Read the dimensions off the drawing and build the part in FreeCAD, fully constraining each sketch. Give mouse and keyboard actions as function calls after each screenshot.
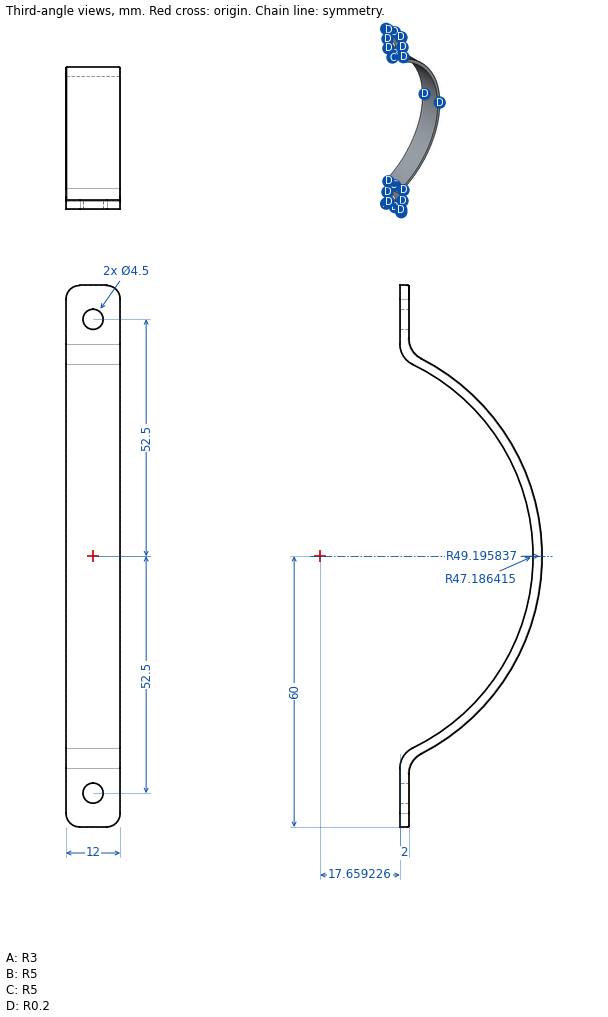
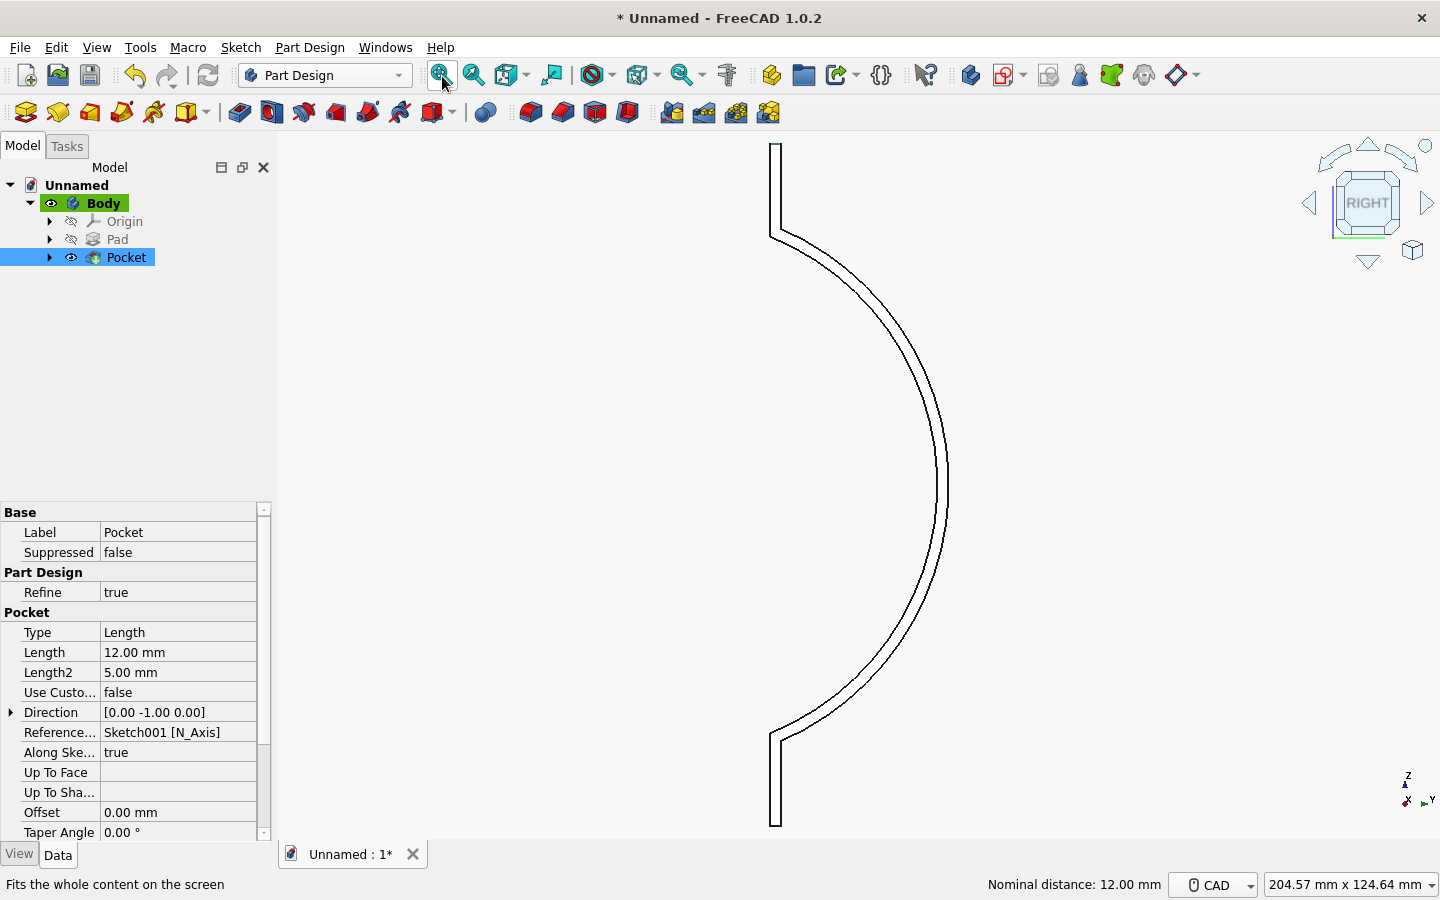
key(5)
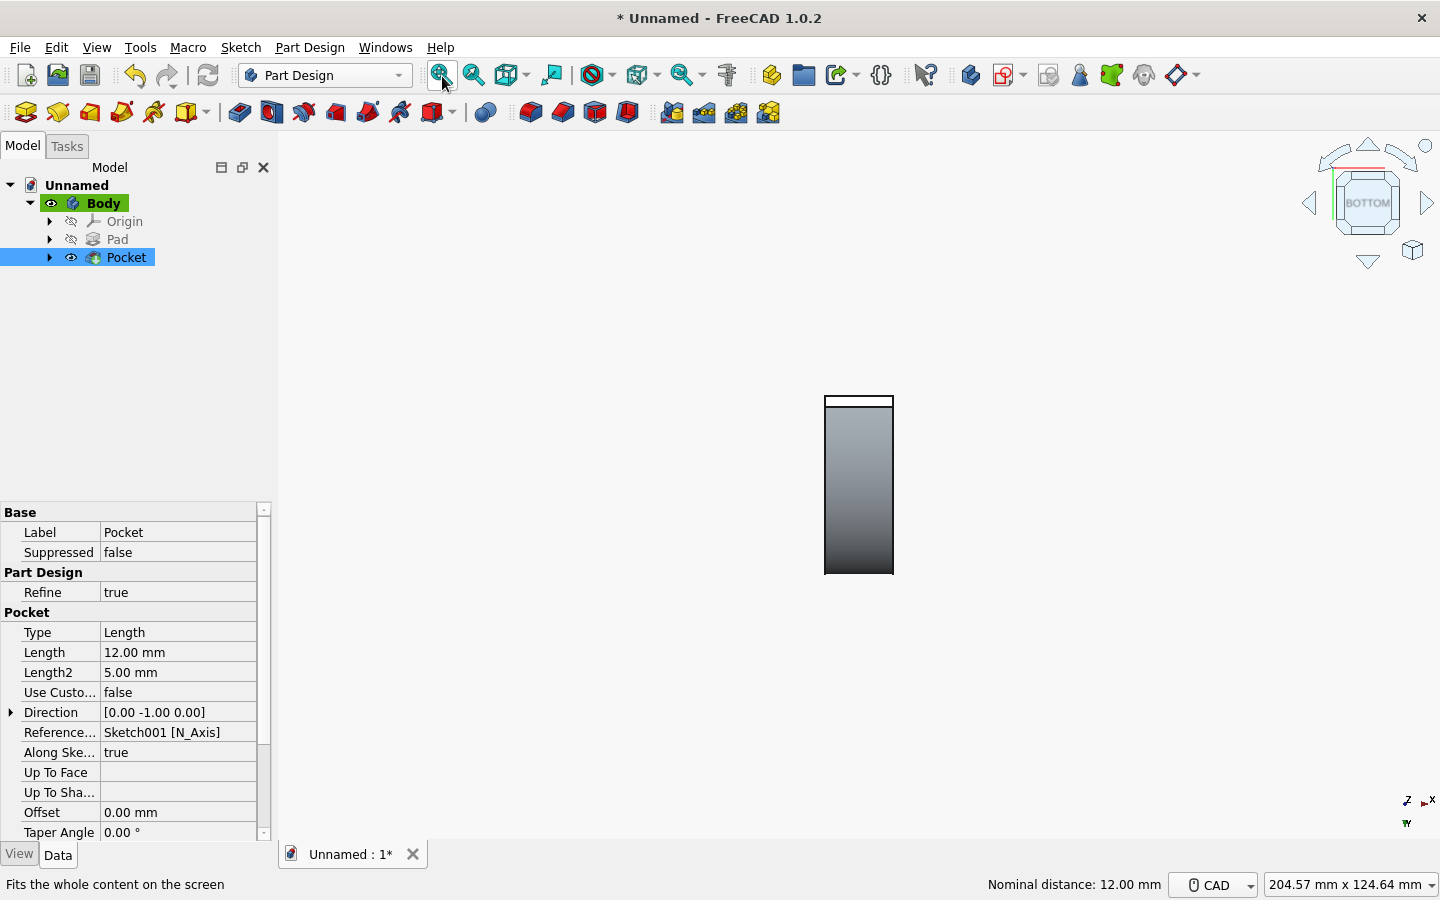
key(v)
key(f)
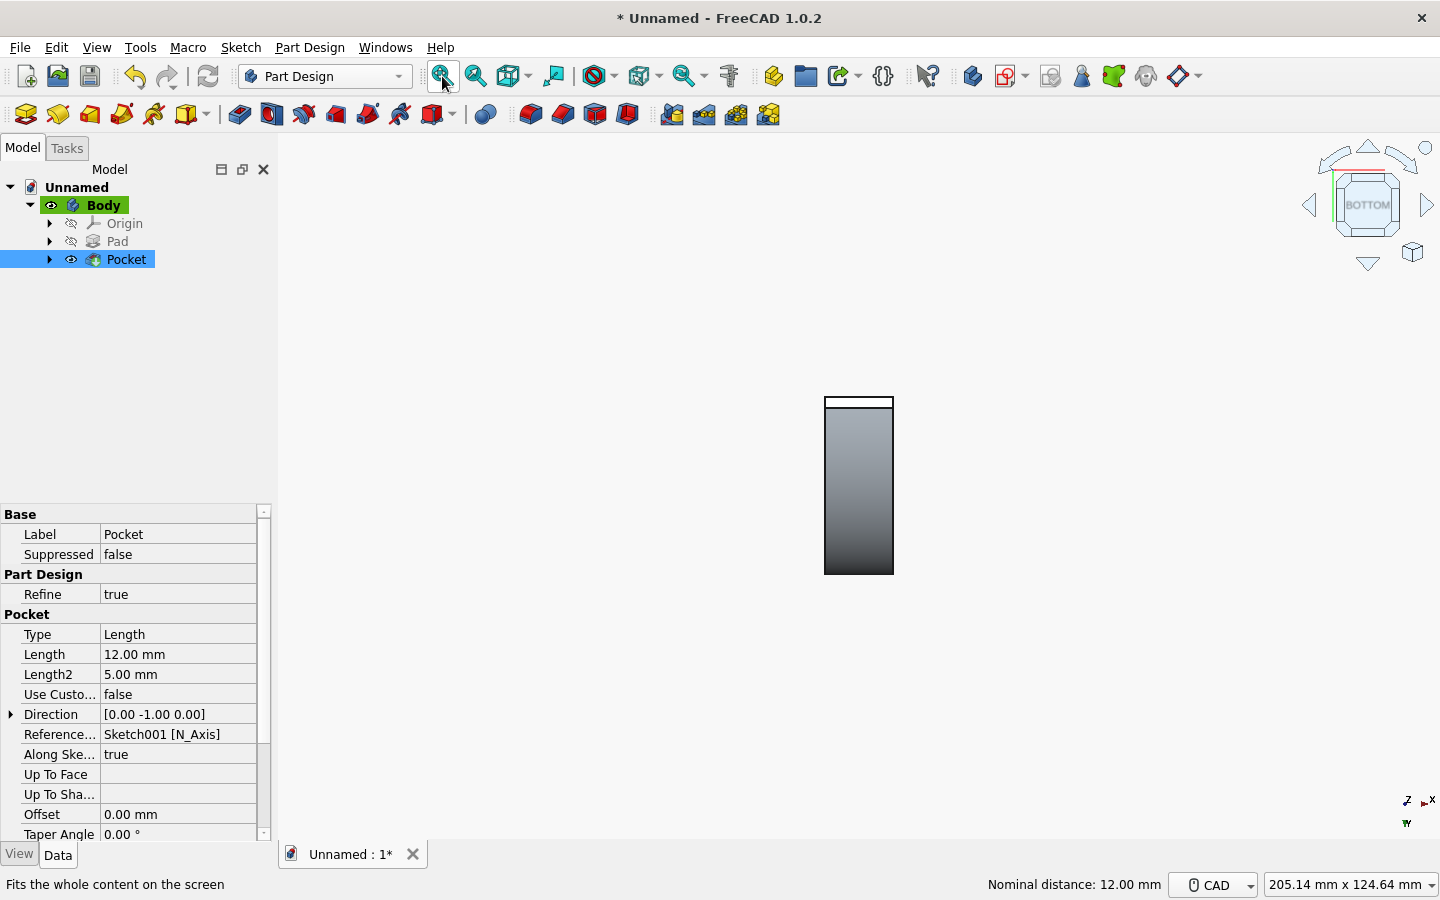
scroll(893, 401, up, 7)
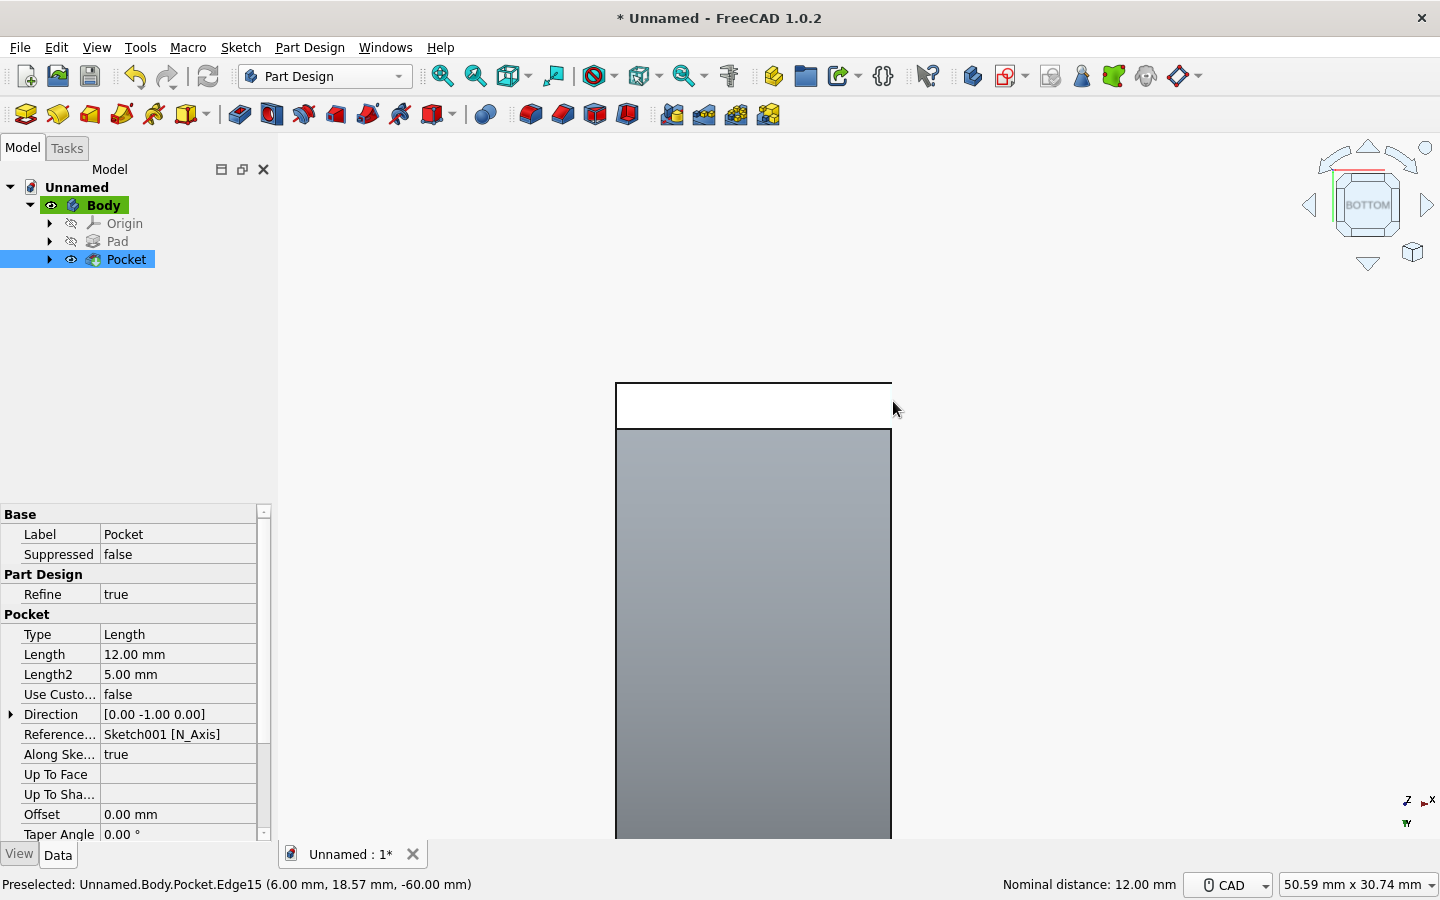
click(891, 405, ctrl)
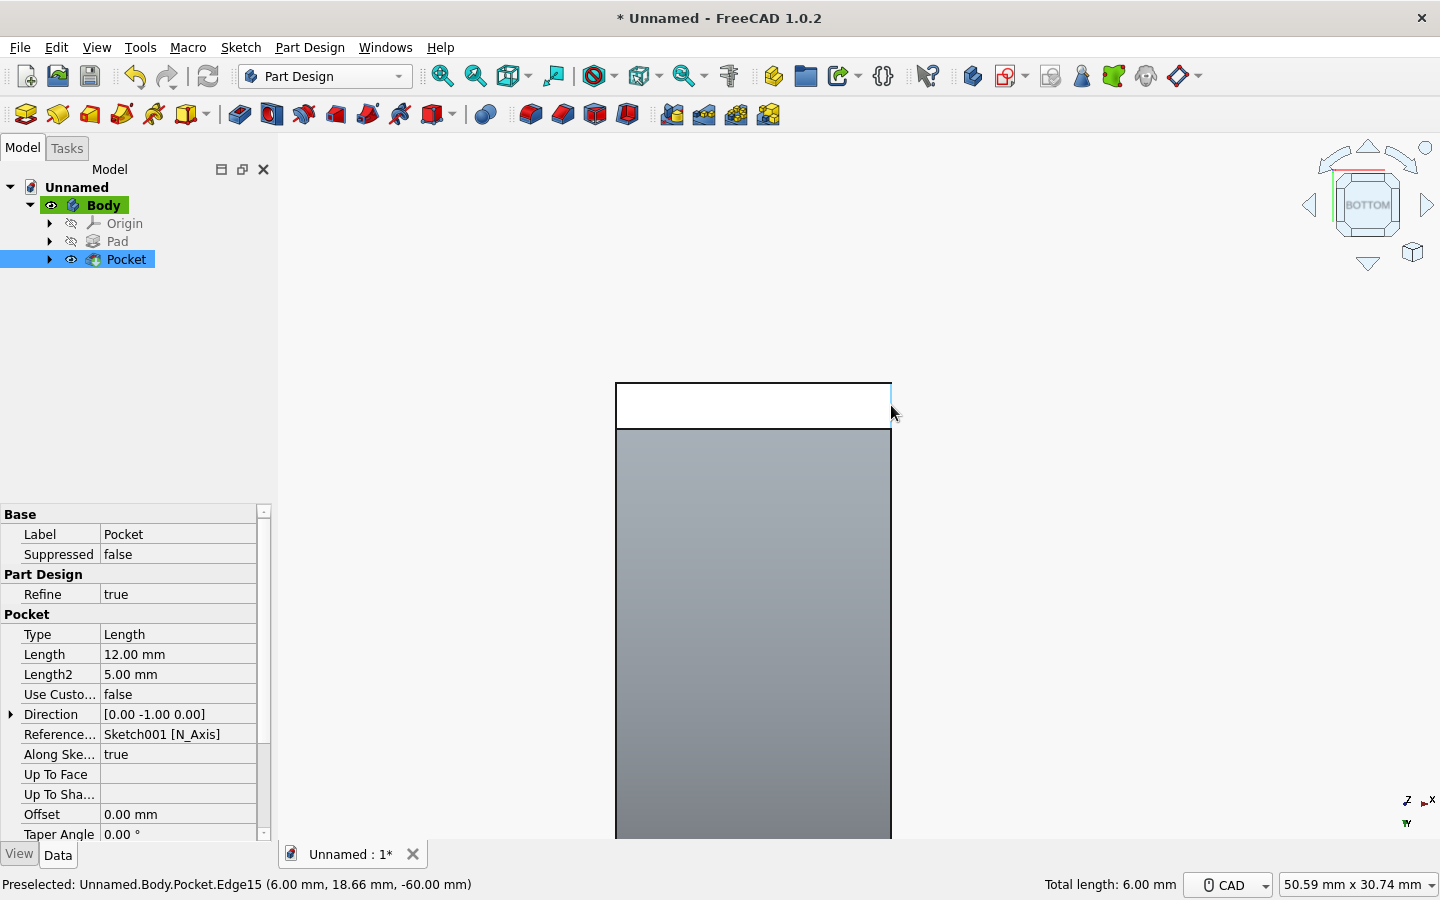
click(616, 405, ctrl)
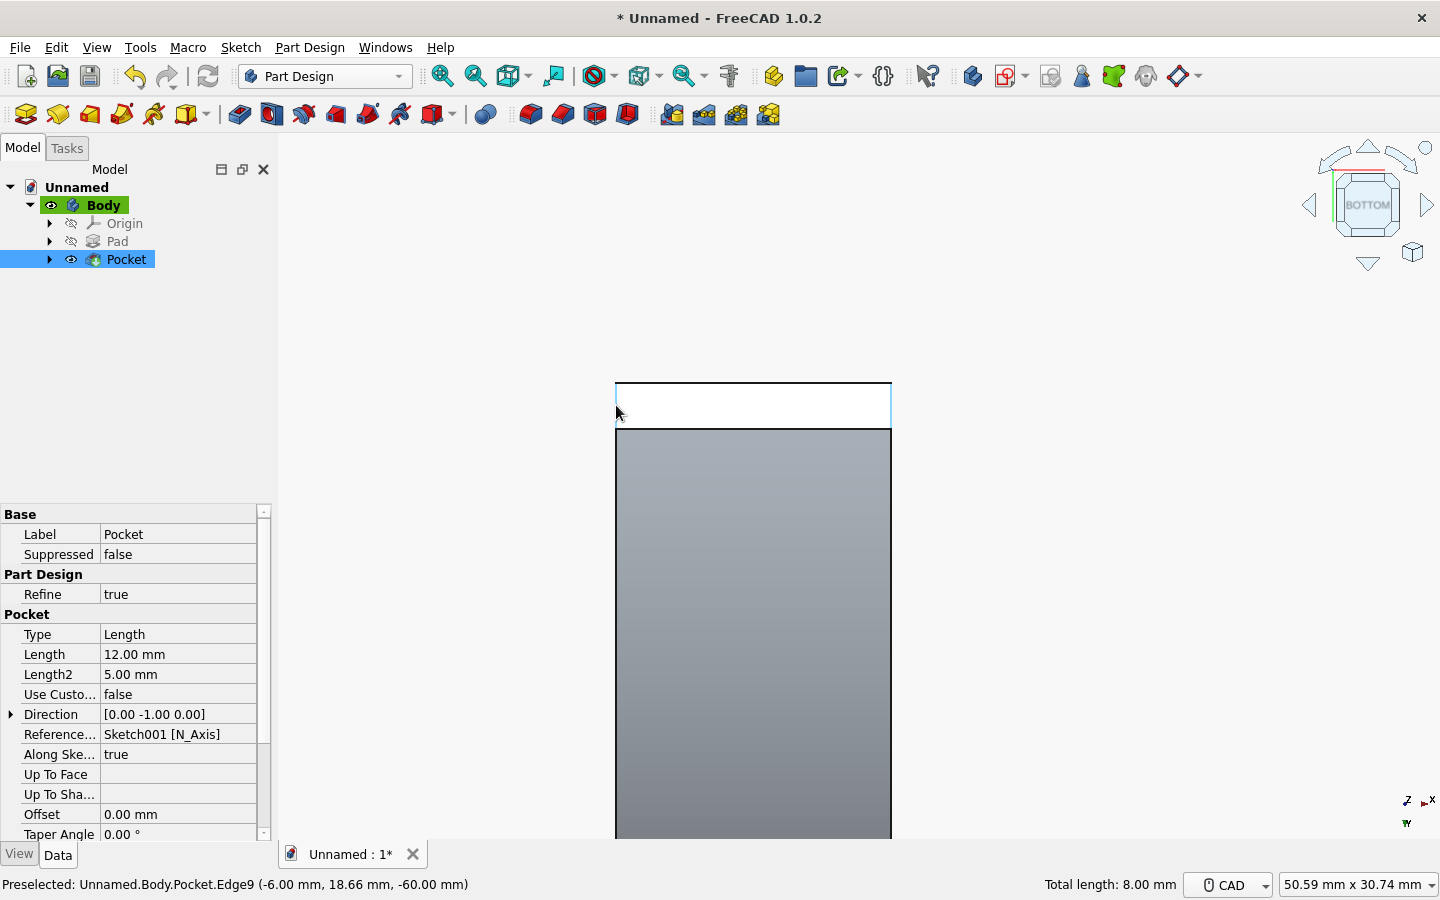
click(532, 114)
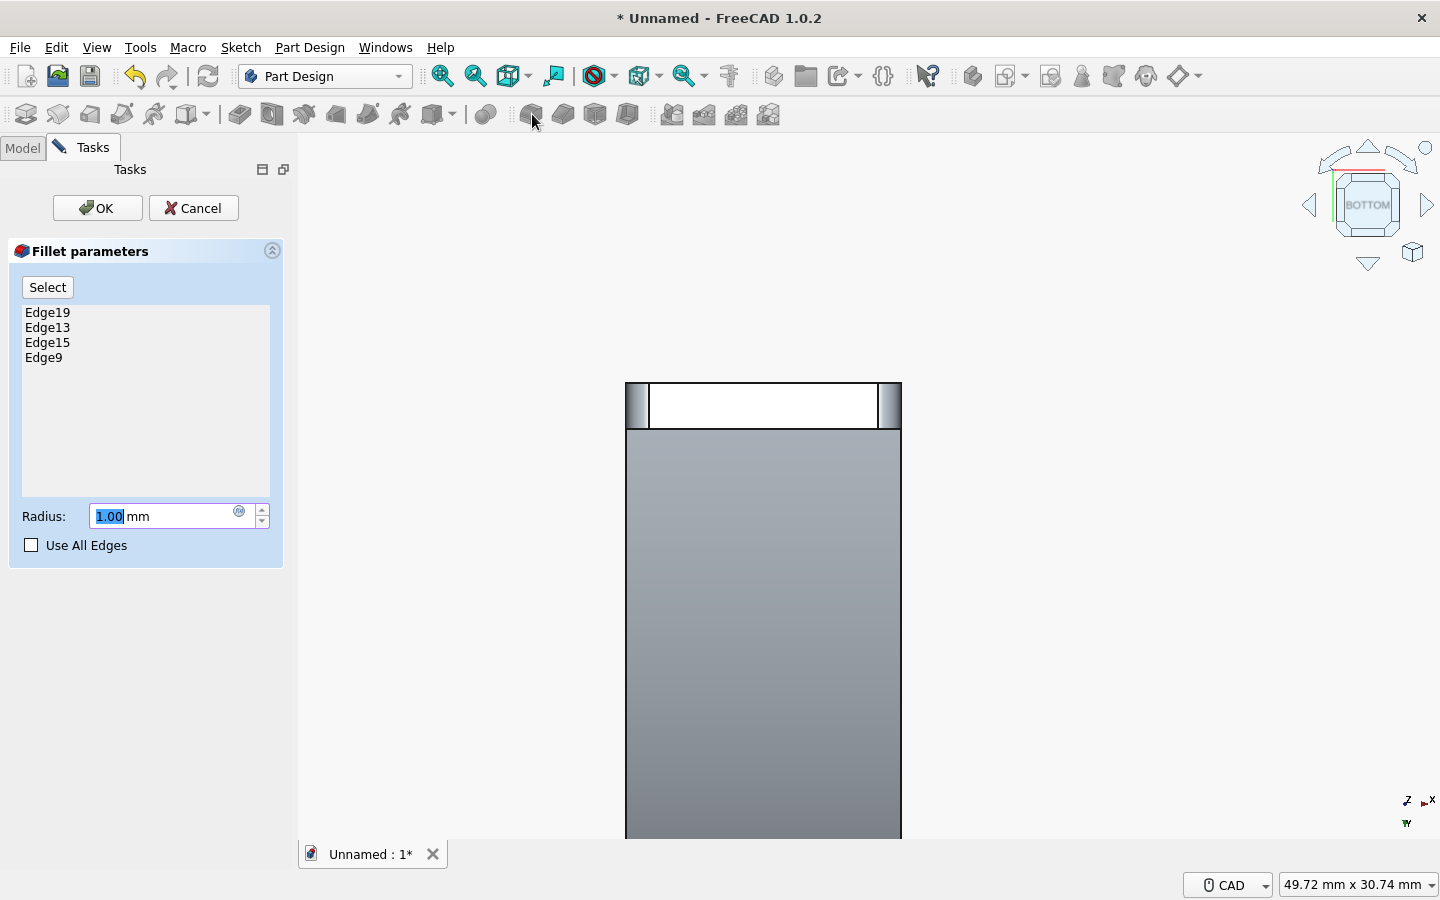
text(3)
key(Tab)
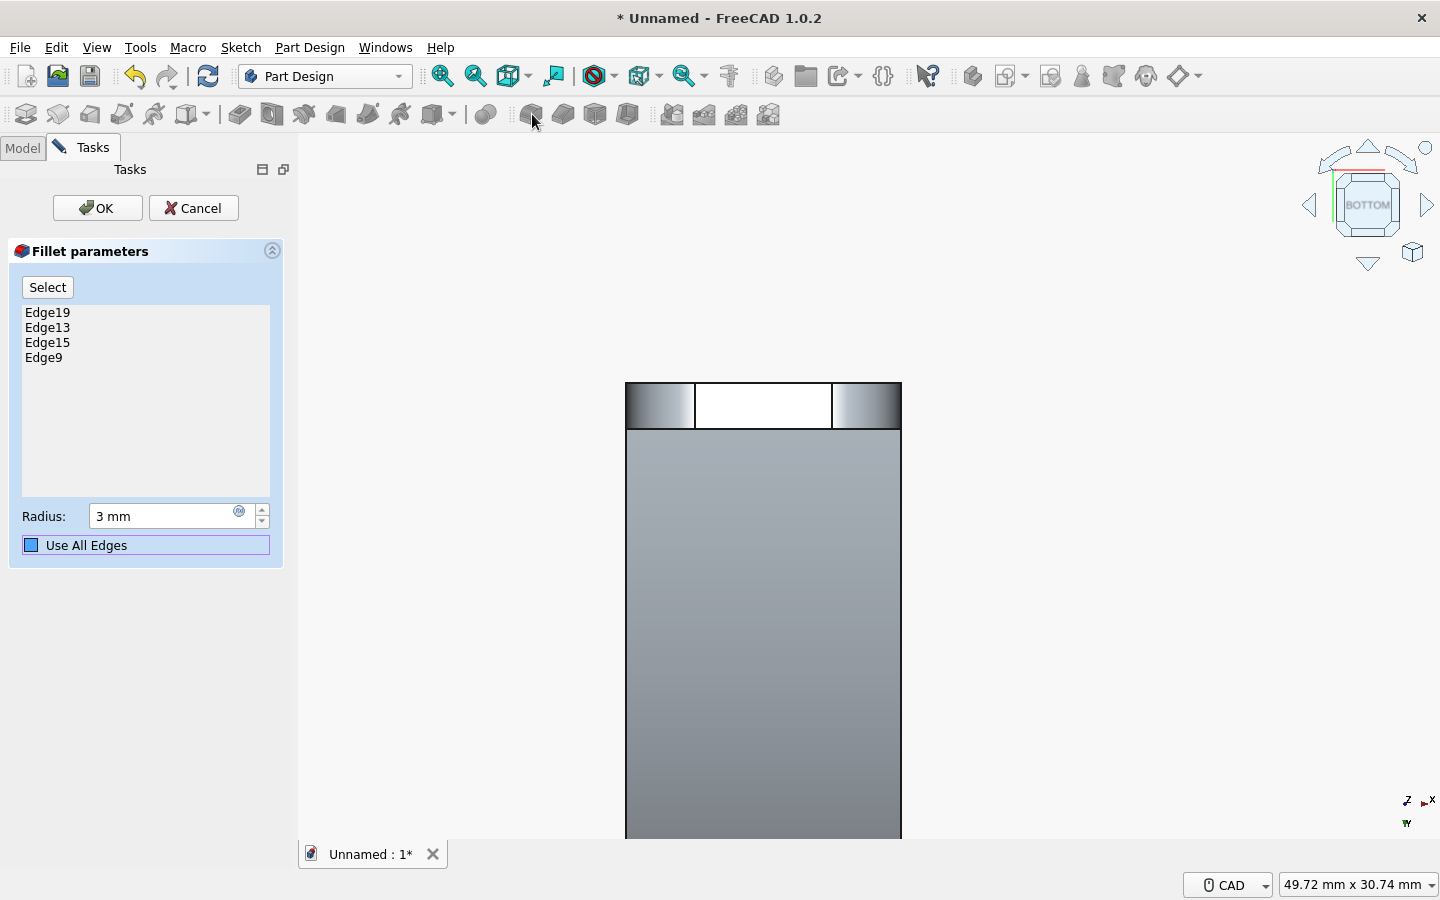
click(98, 208)